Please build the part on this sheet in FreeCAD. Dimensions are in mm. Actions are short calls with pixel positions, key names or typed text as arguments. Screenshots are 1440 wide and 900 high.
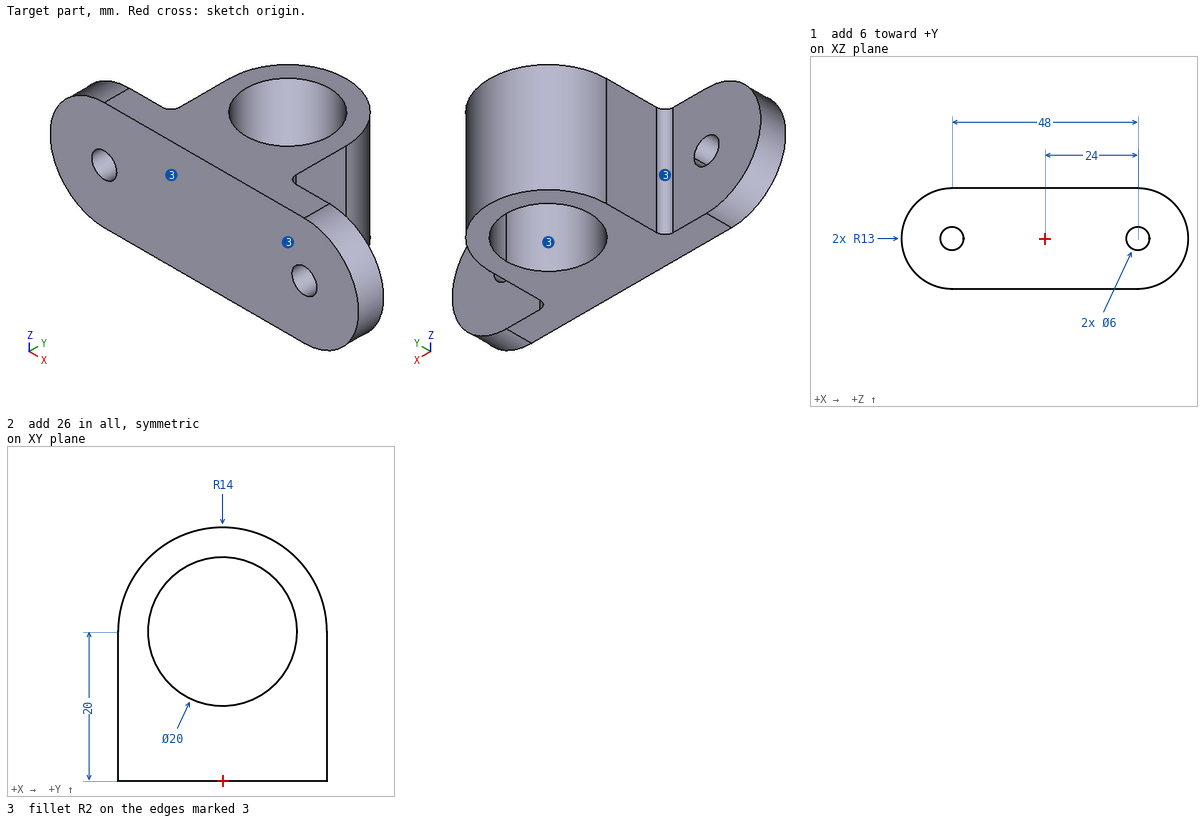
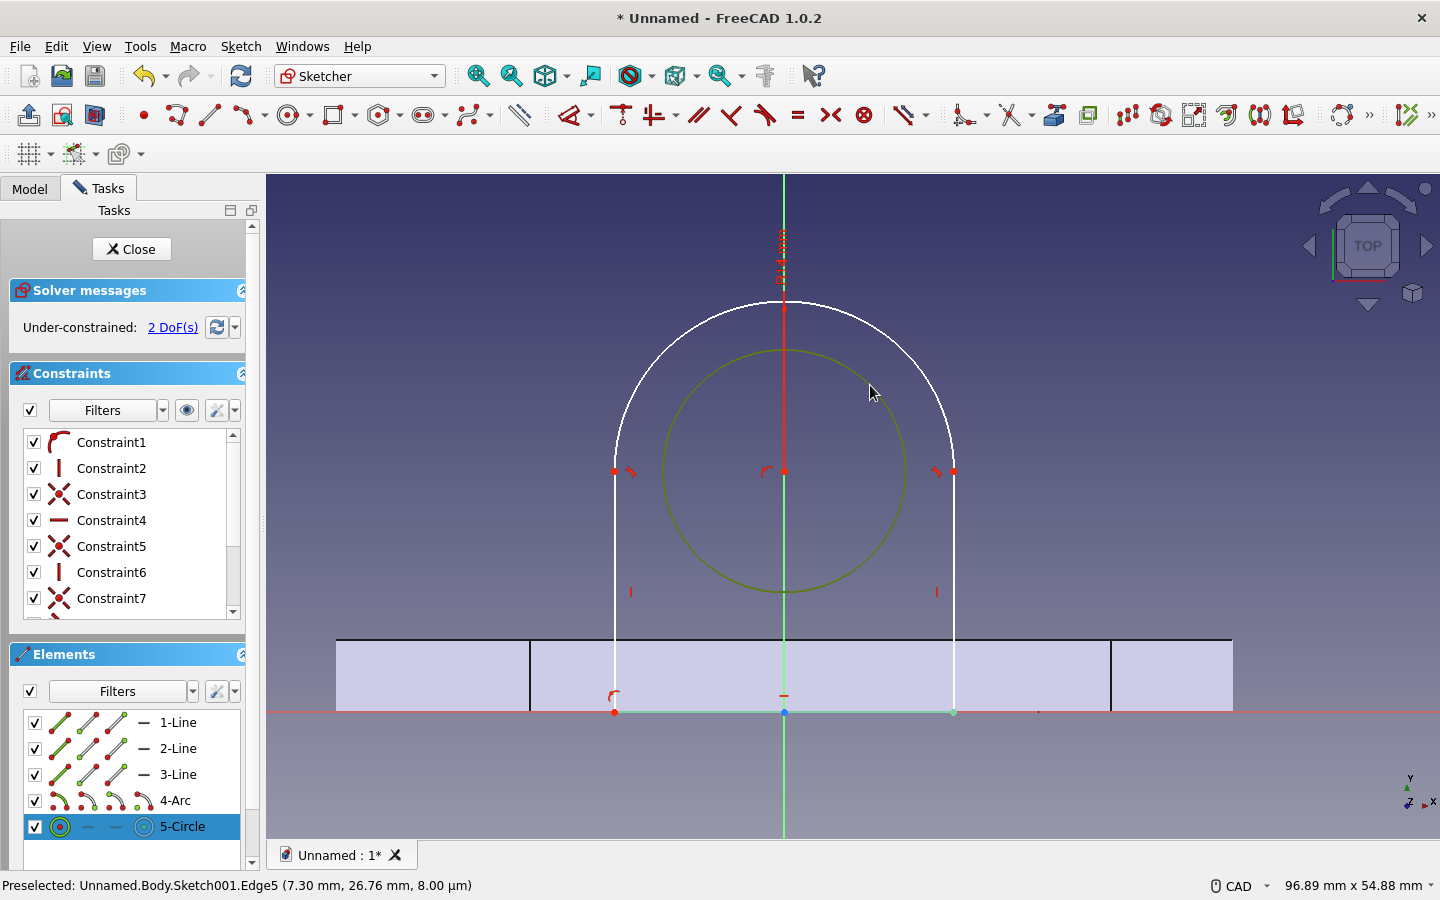
key(k)
key(o)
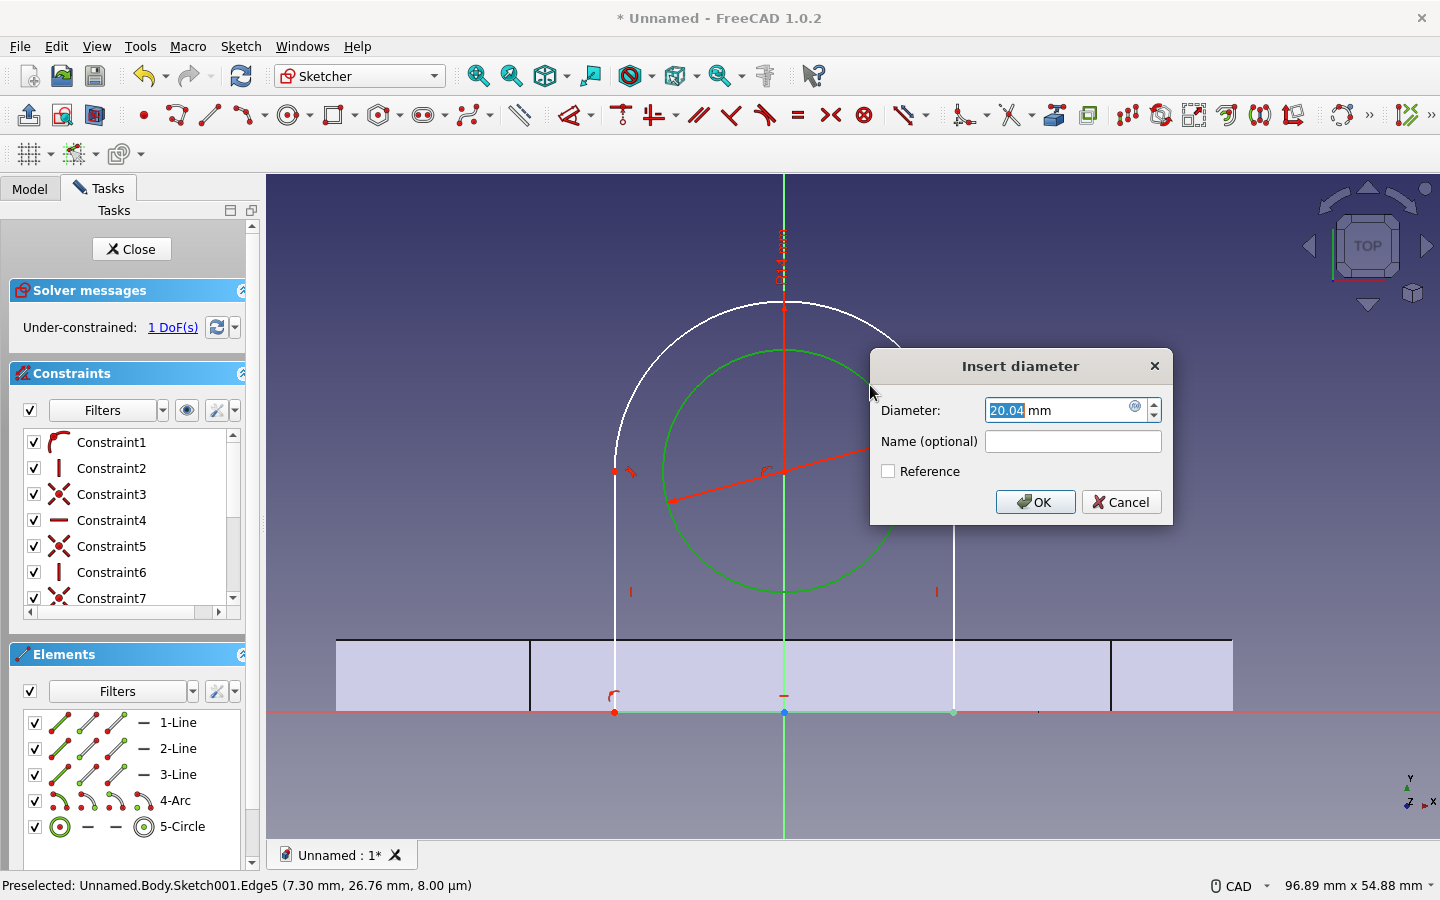
text(20)
key(Return)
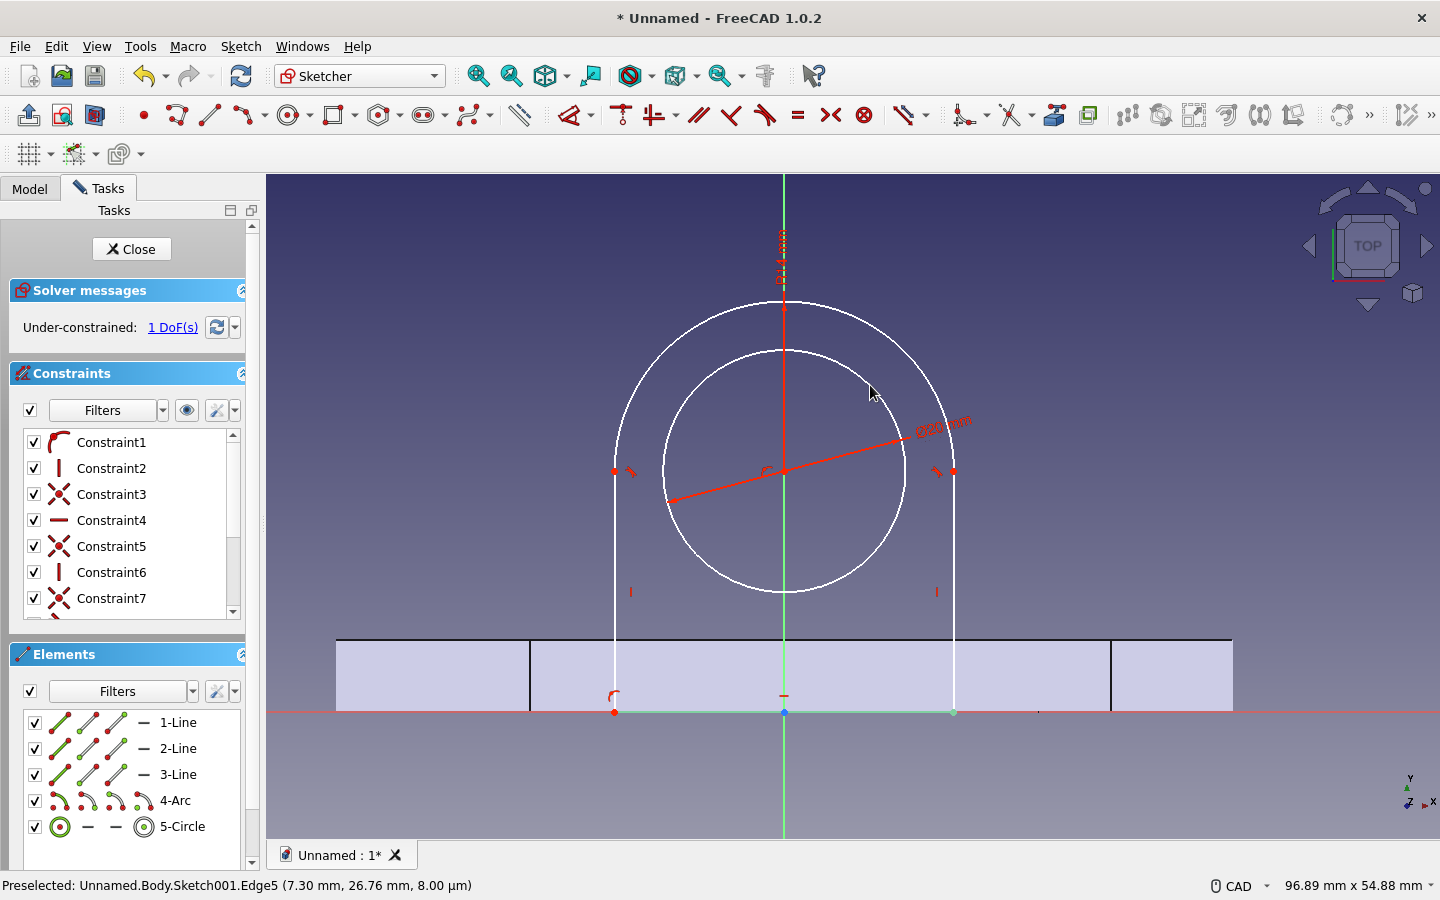
click(615, 544)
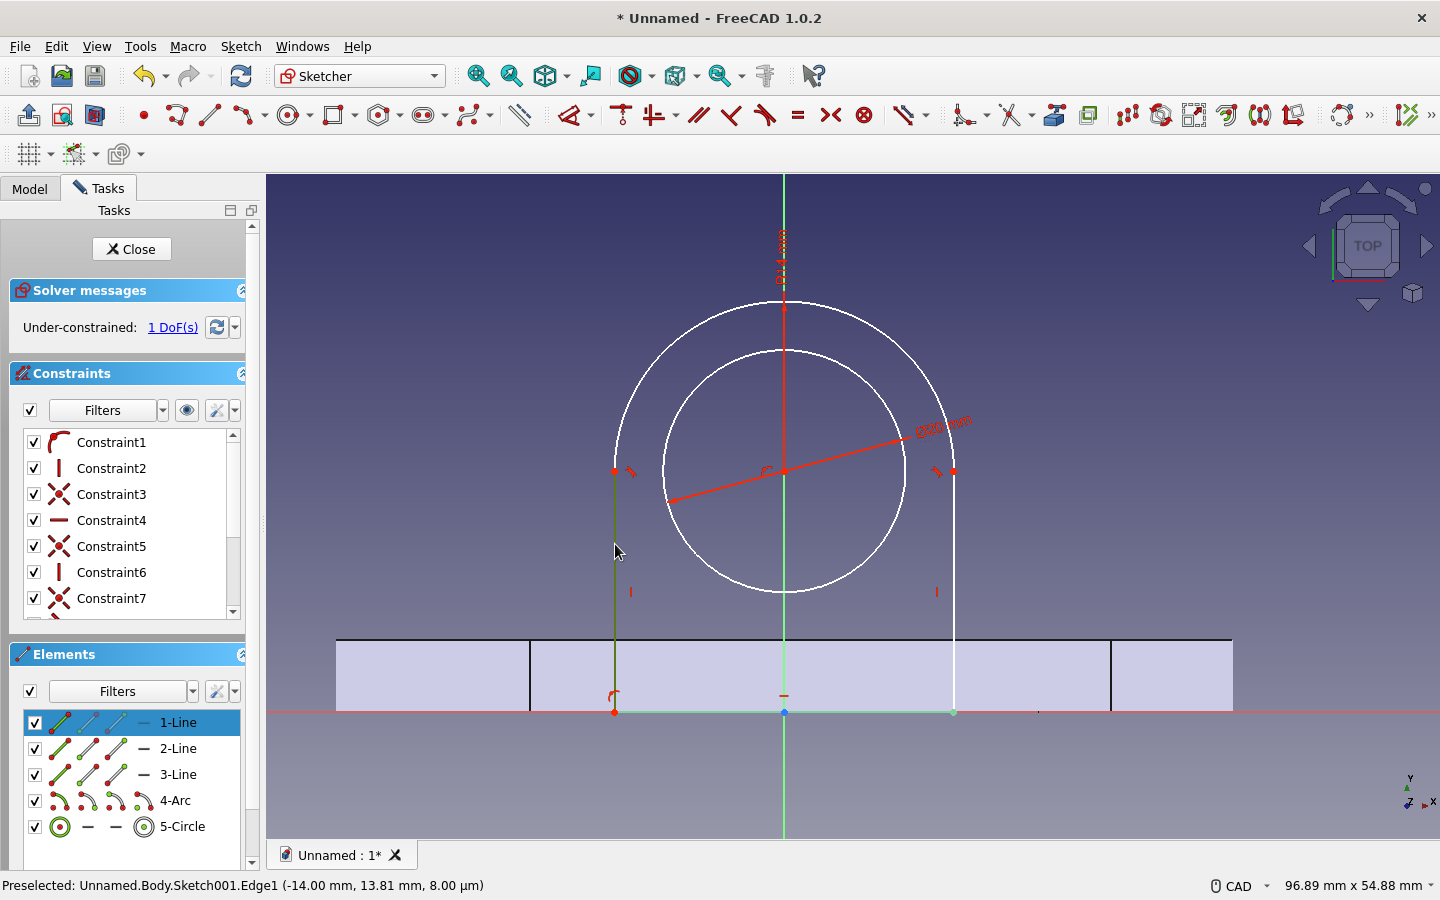
key(i)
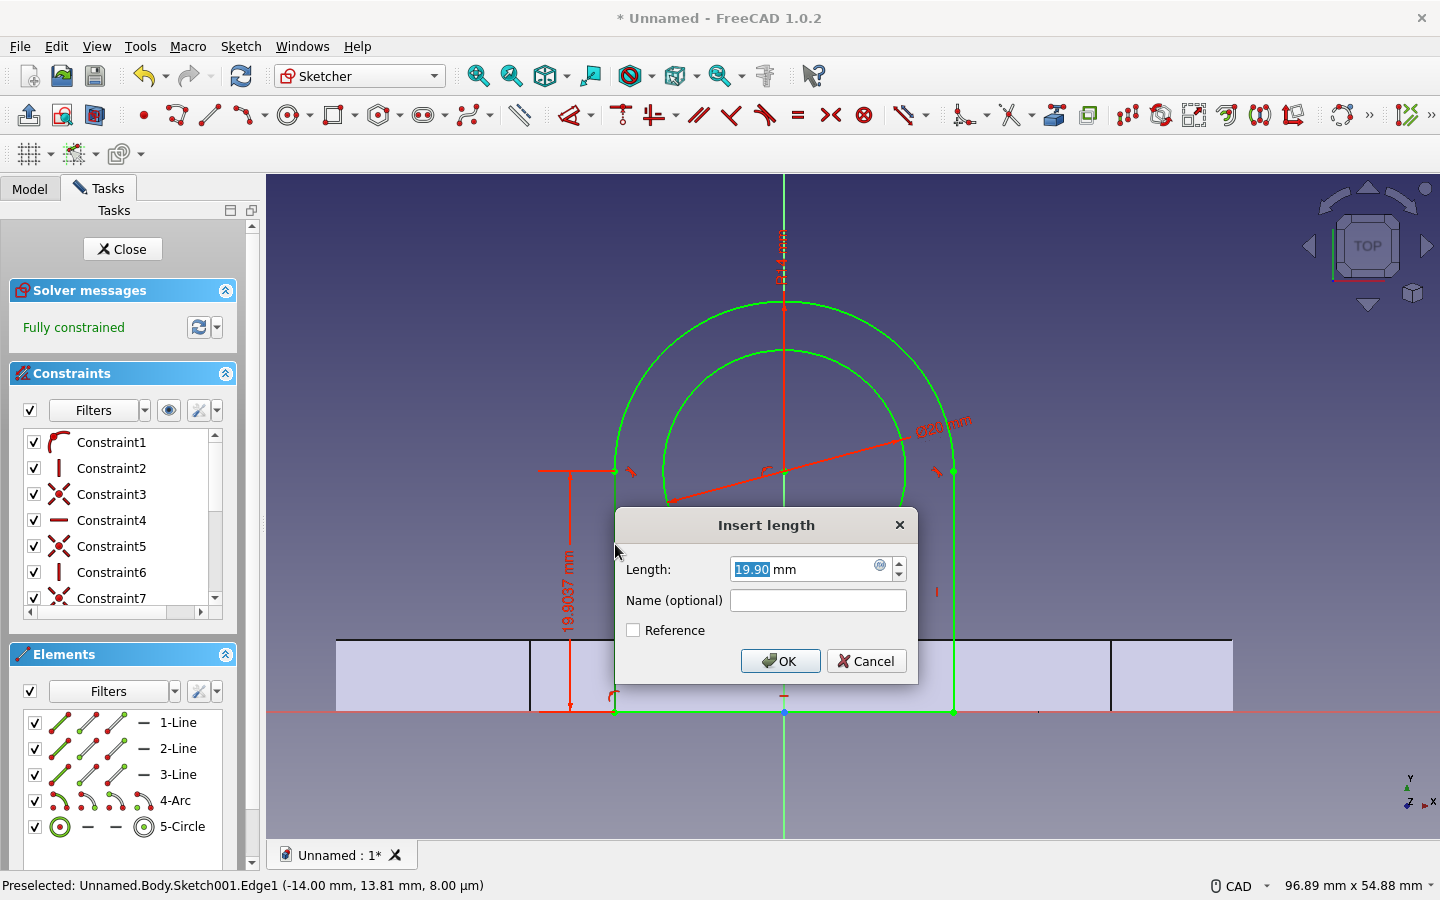
text(20)
key(Return)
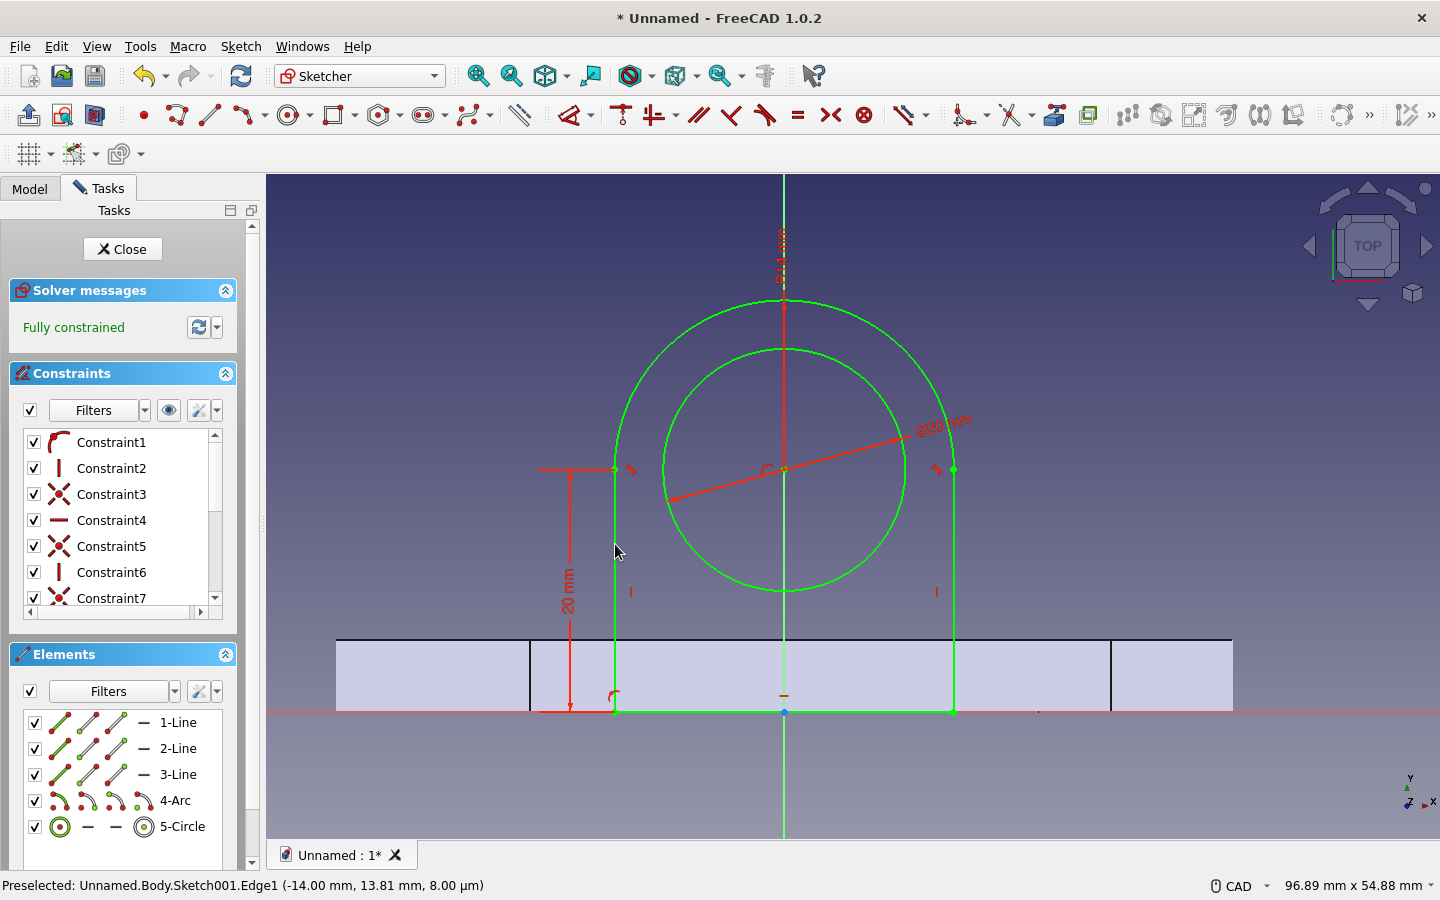
click(123, 249)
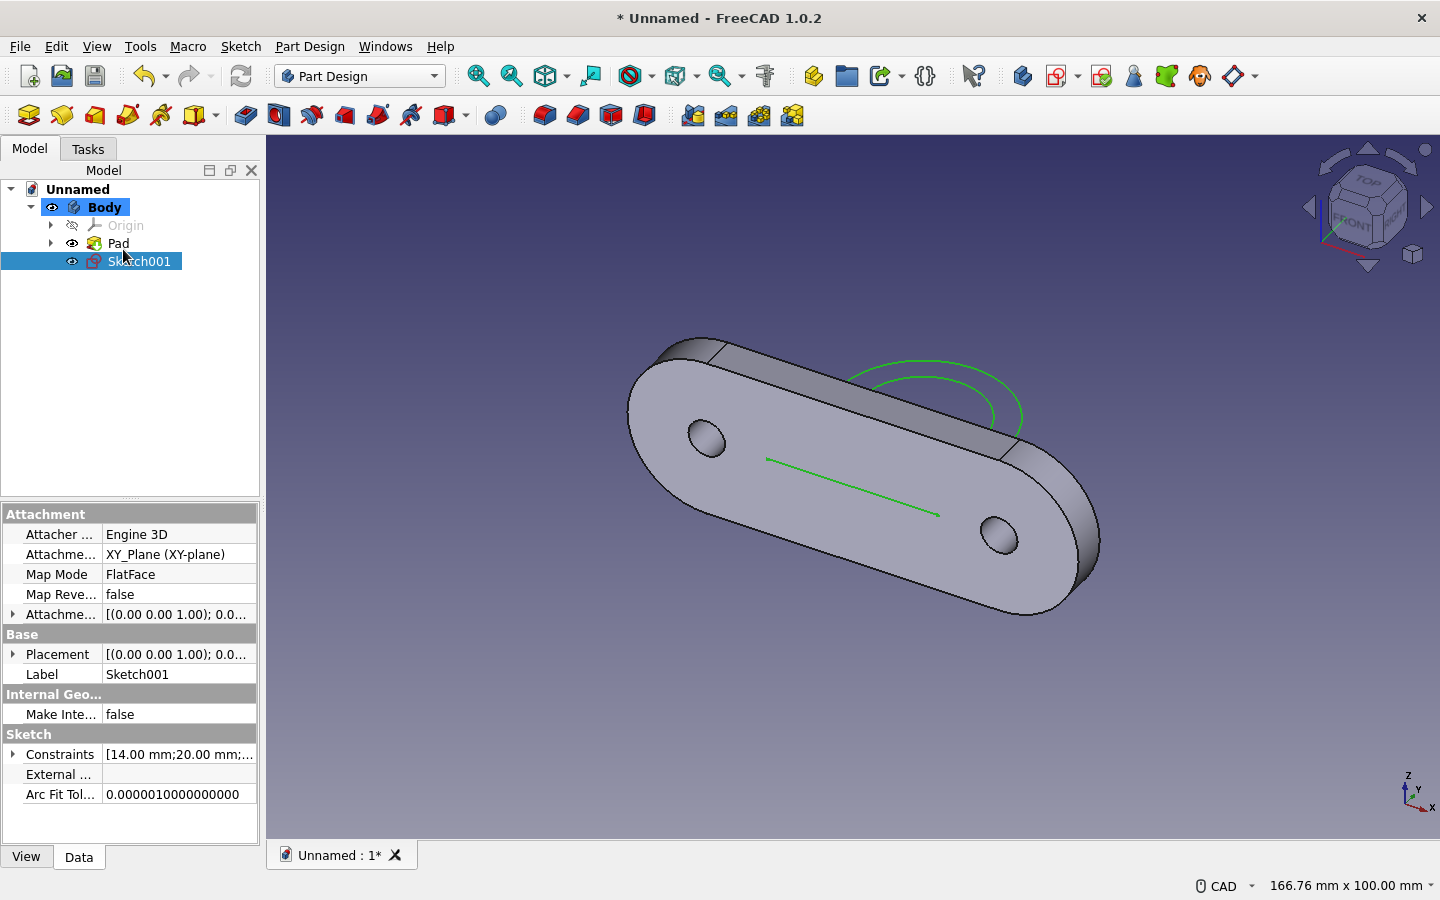
click(29, 116)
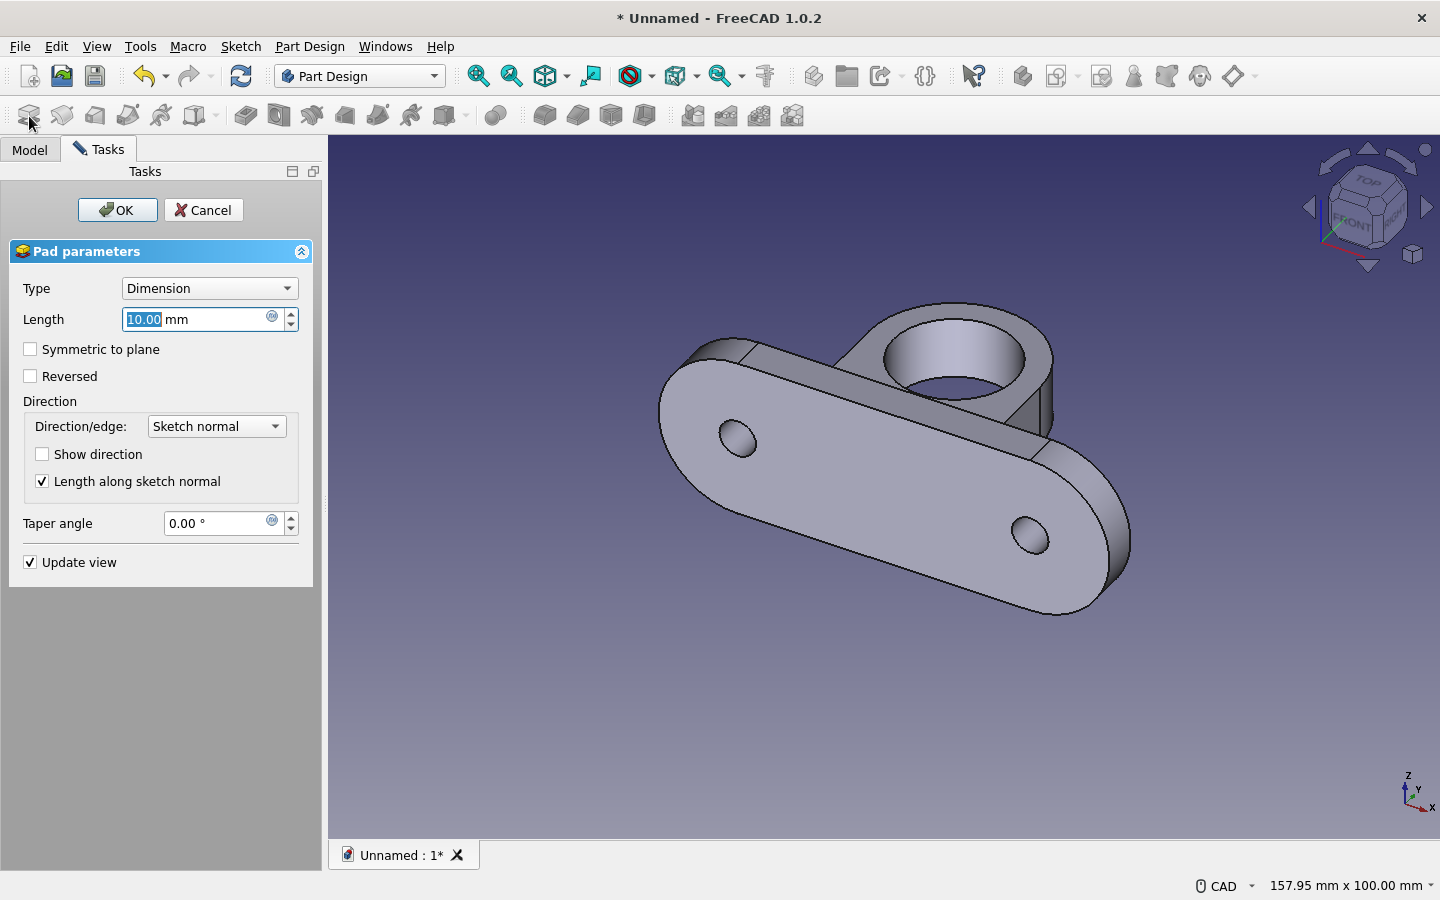
text(26)
key(Tab)